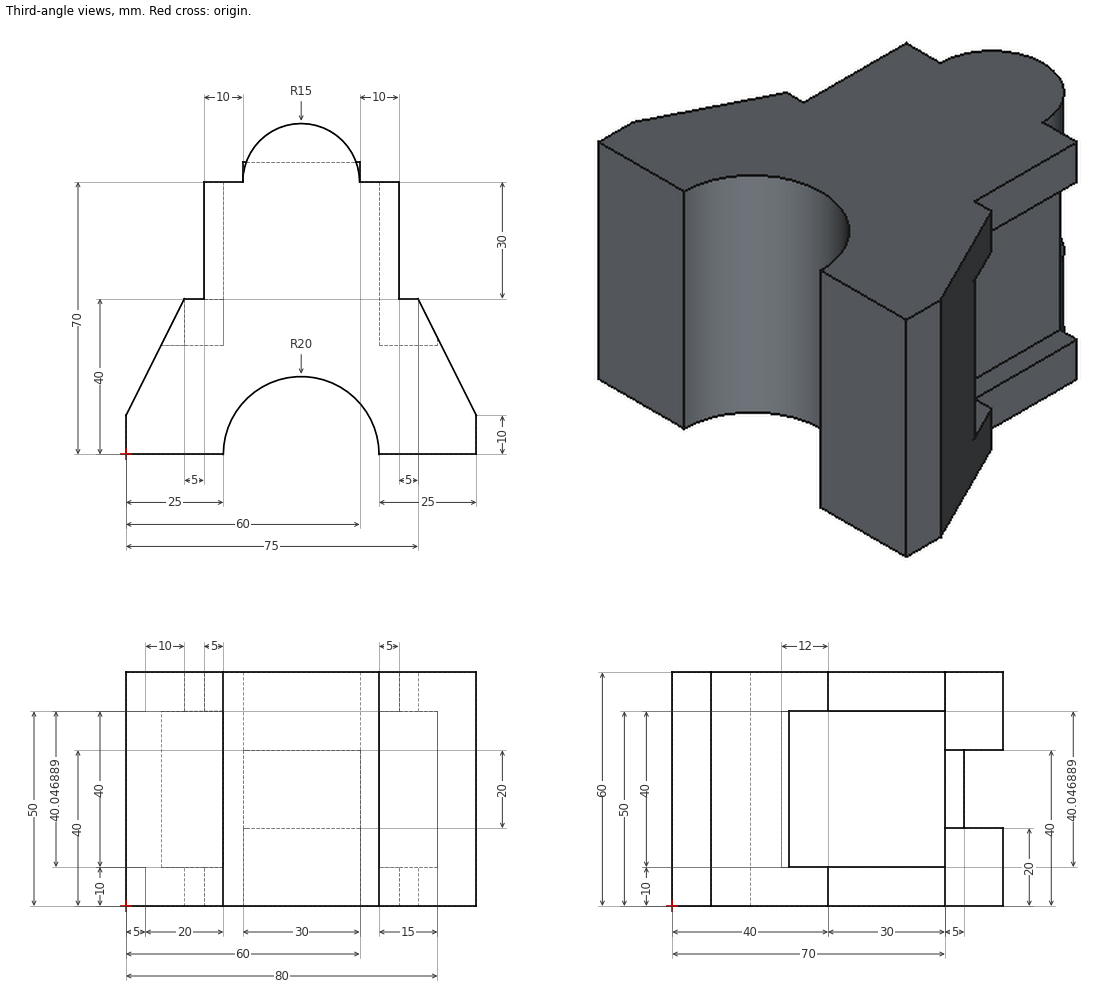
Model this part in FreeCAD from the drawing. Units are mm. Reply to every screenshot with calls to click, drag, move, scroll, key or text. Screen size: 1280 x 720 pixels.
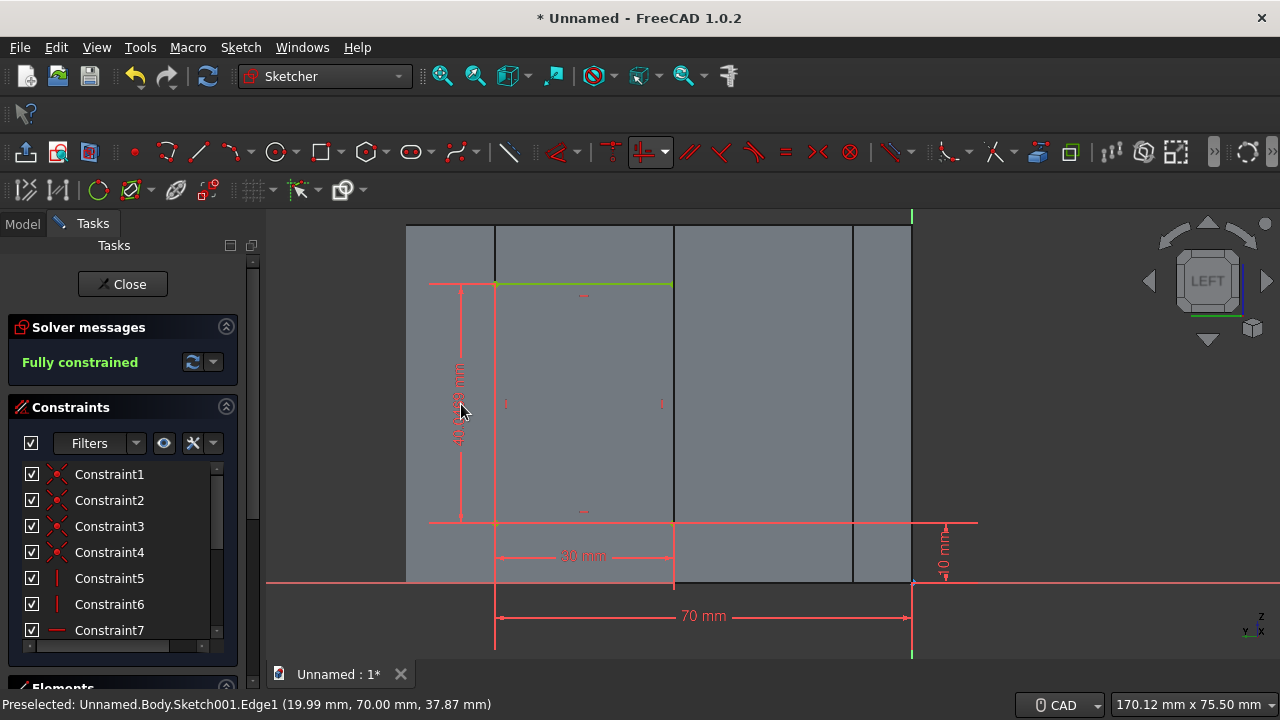
click(123, 284)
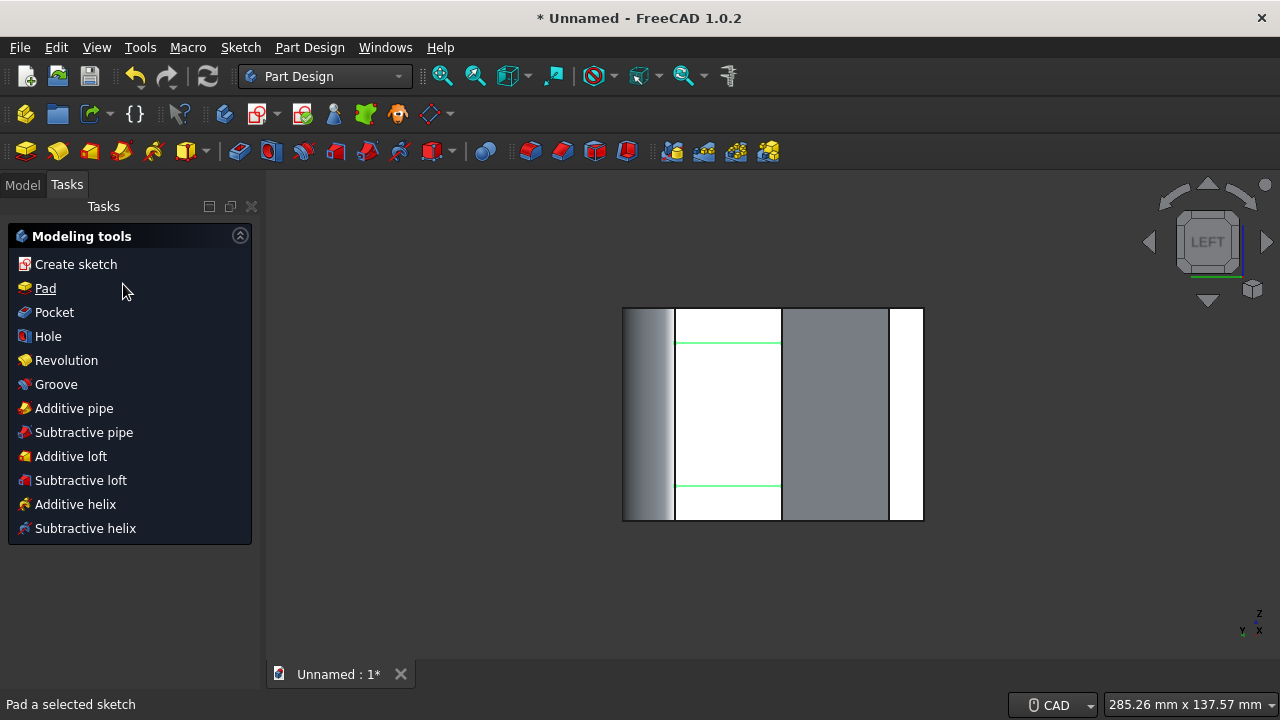
click(240, 152)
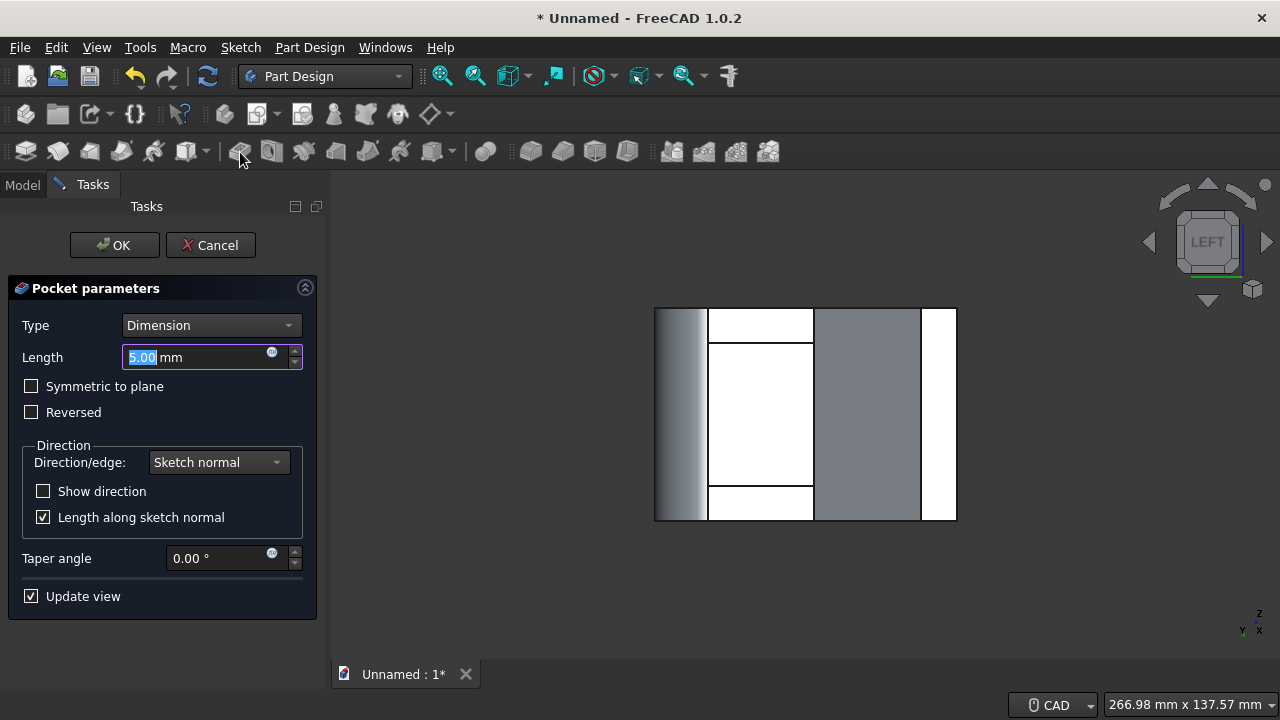
text(5)
key(Tab)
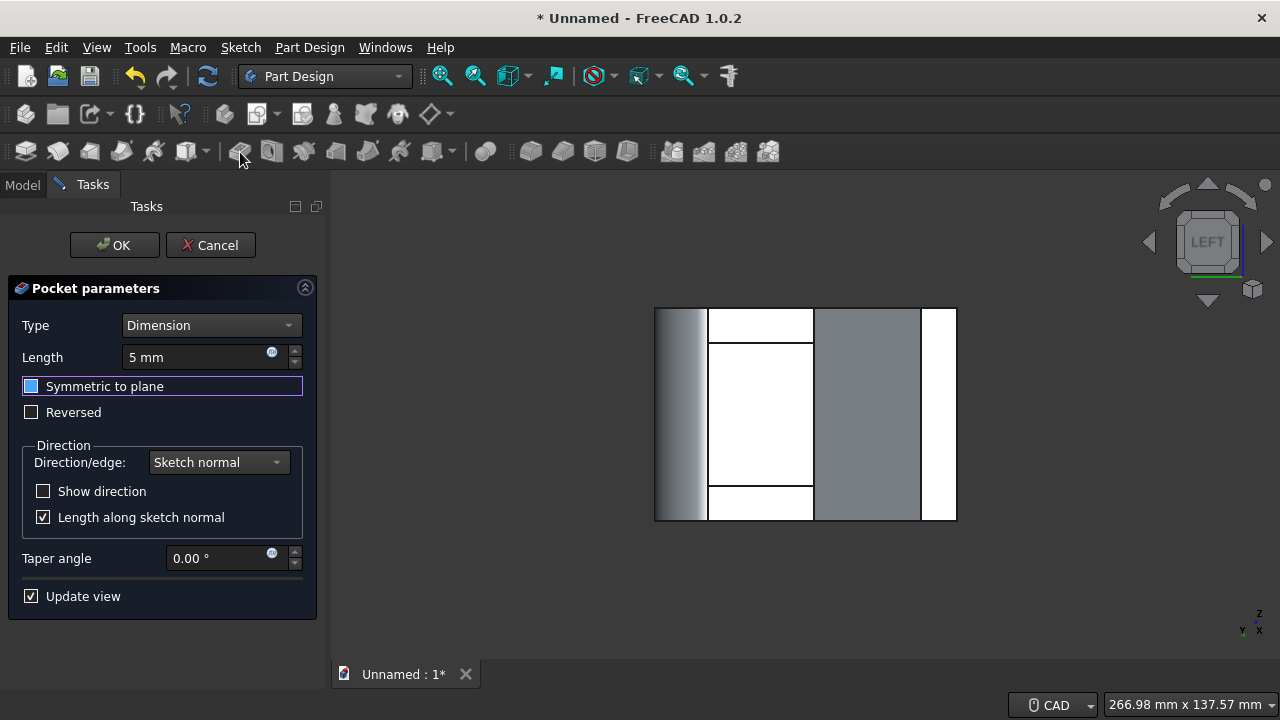
click(115, 245)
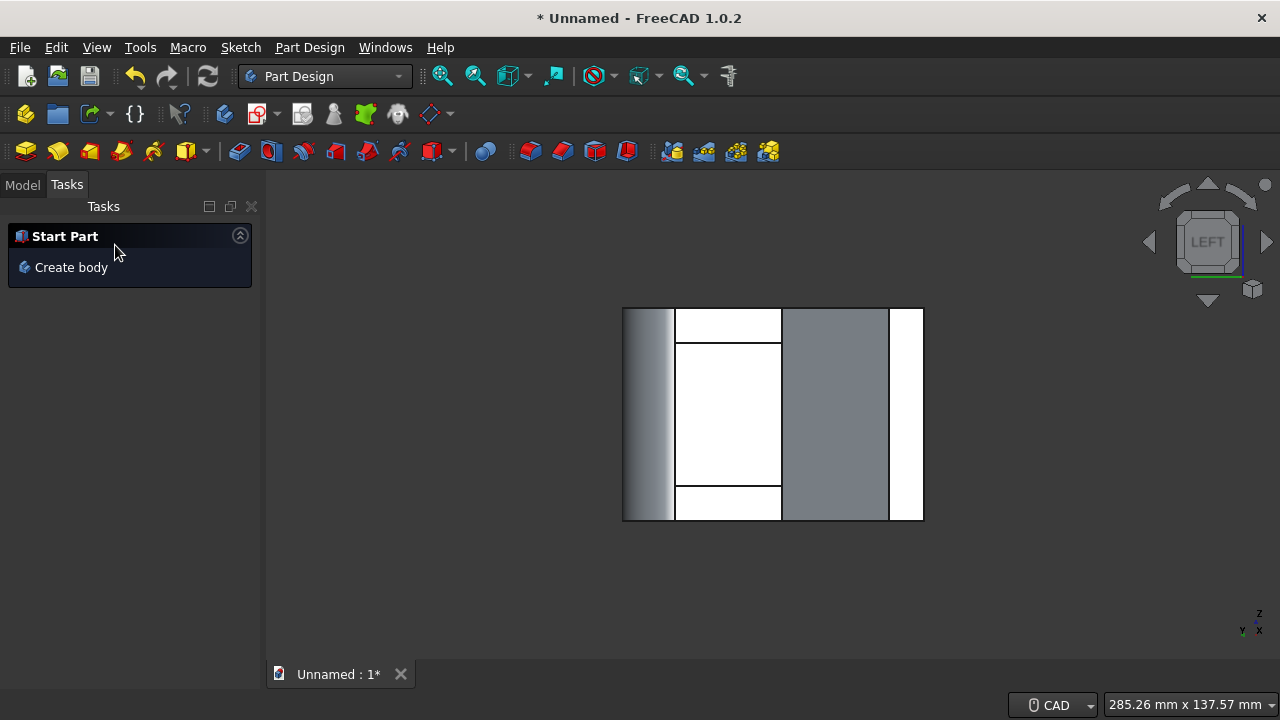
key(v)
key(f)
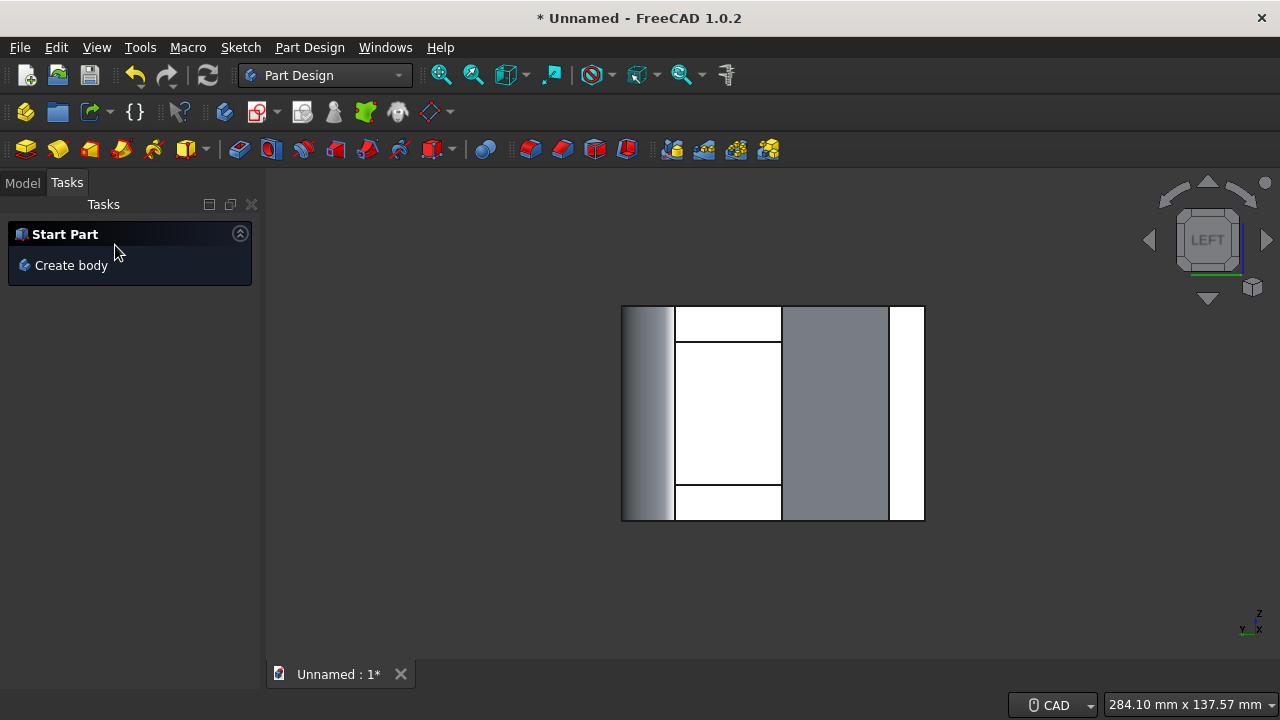
key(4)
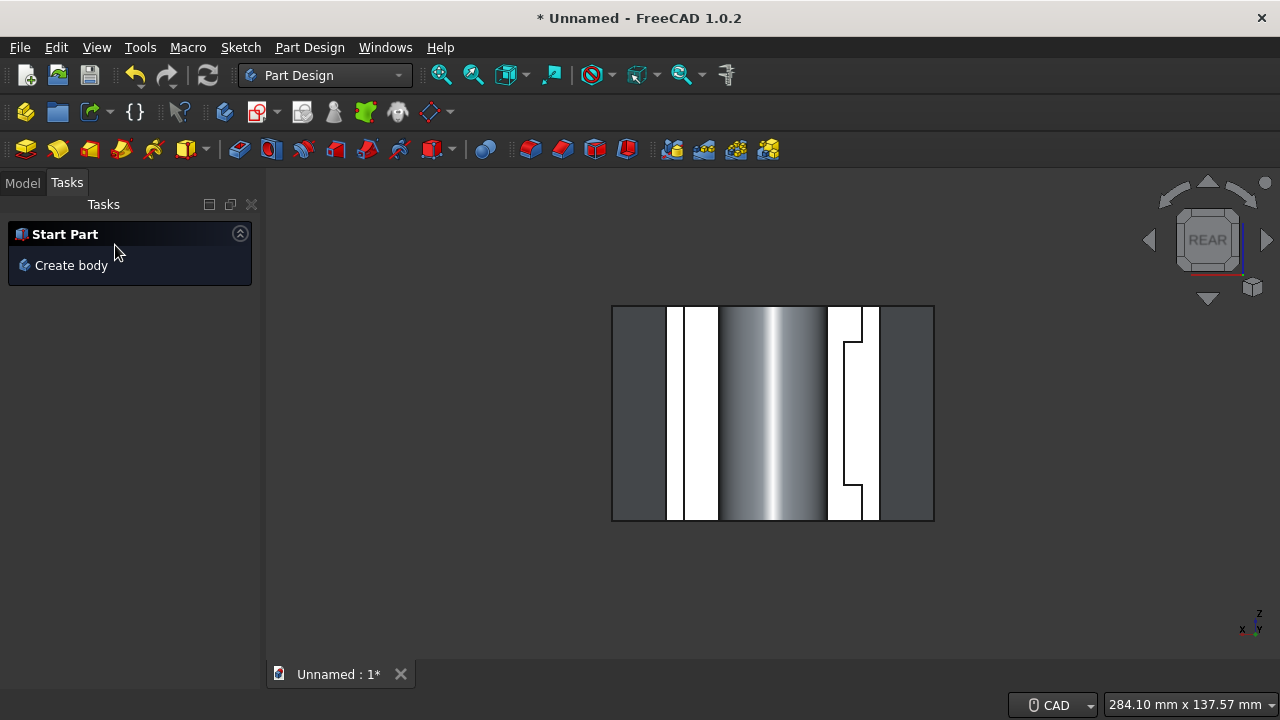
key(v)
key(f)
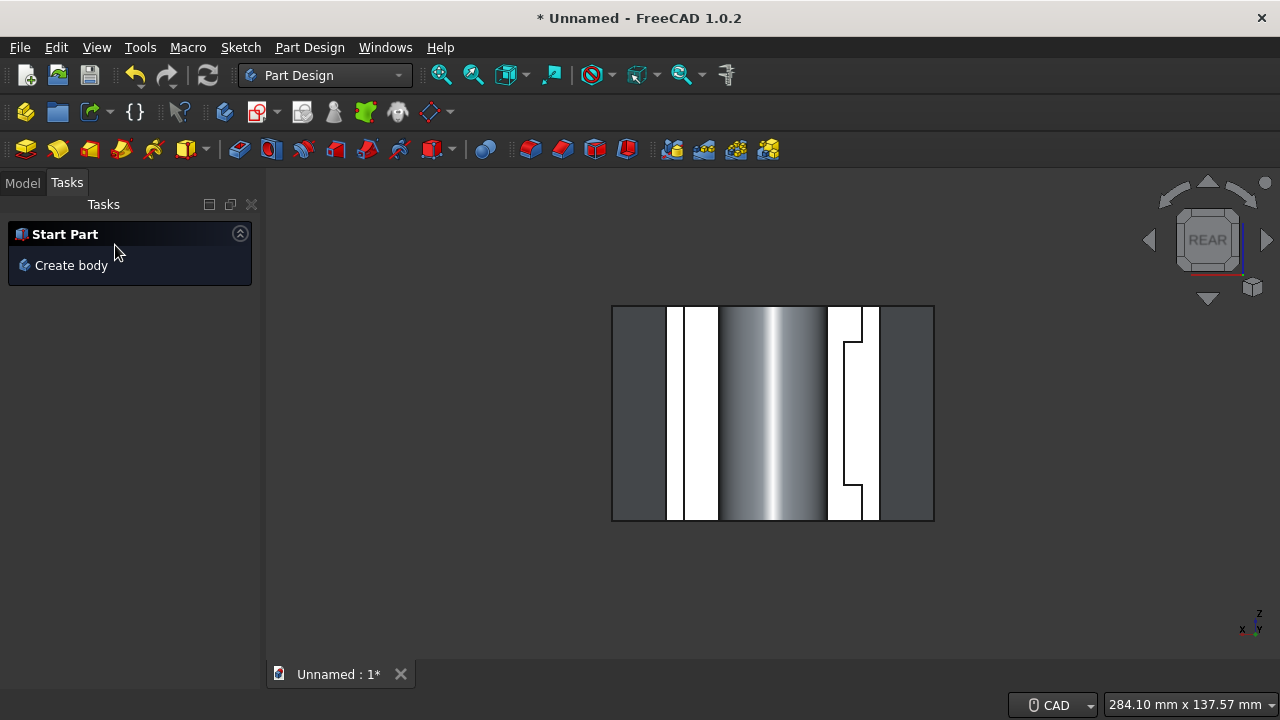
click(862, 382)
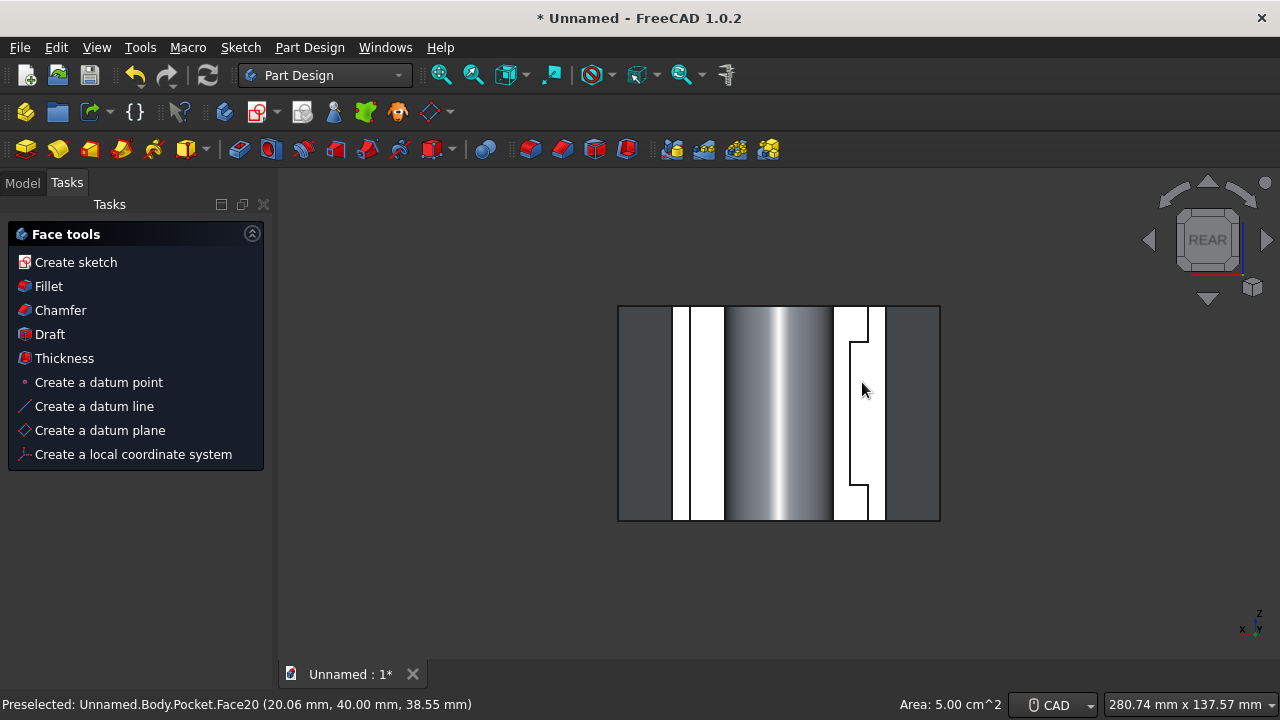
click(258, 112)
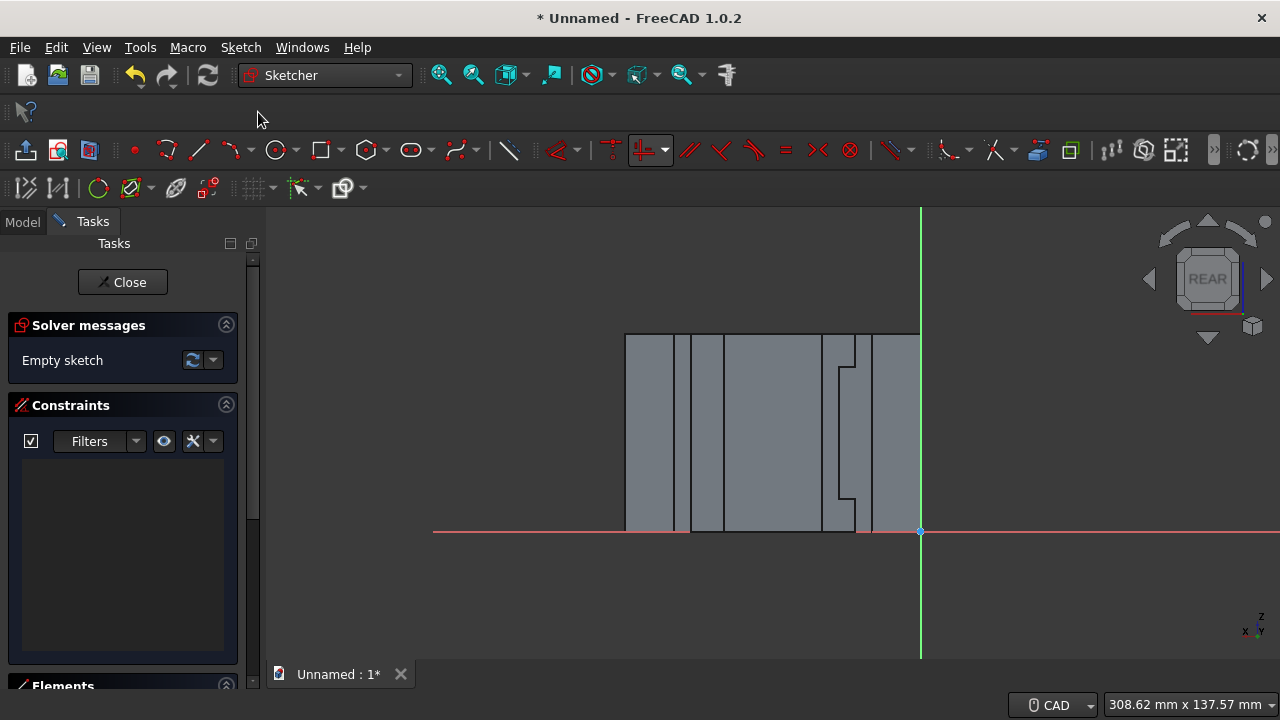
key(q)
key(s)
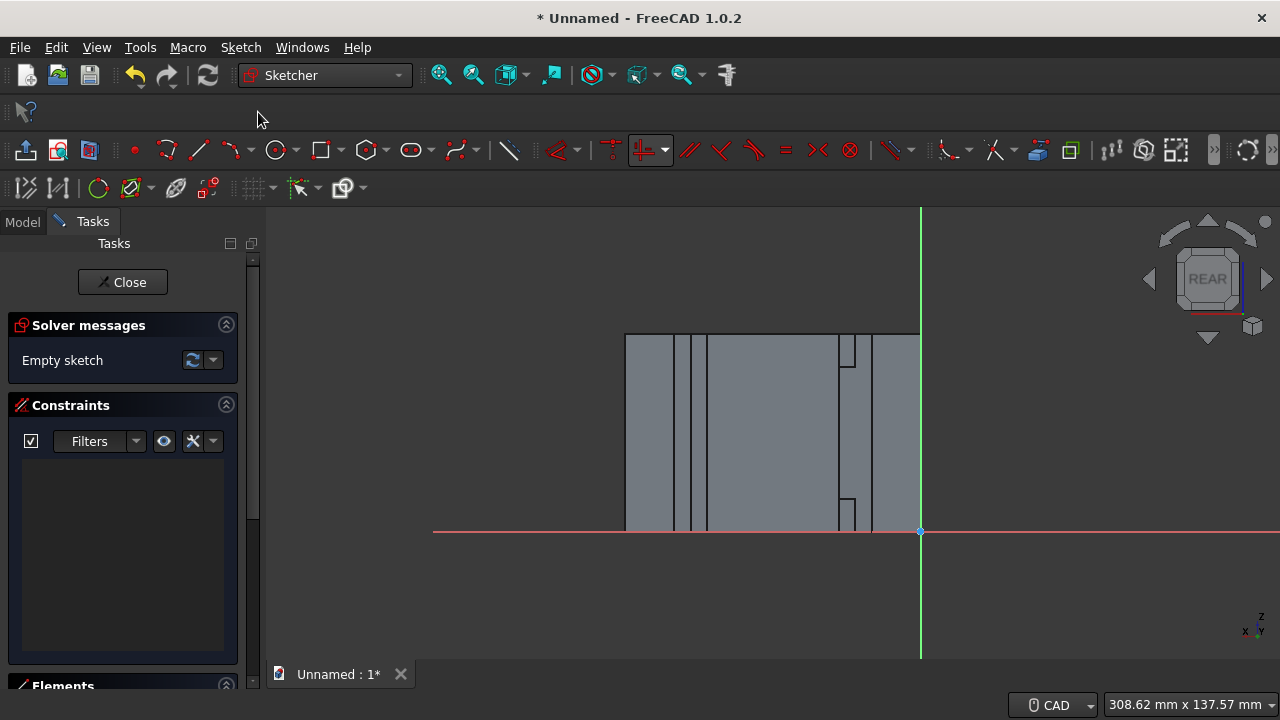
scroll(1093, 469, up, 3)